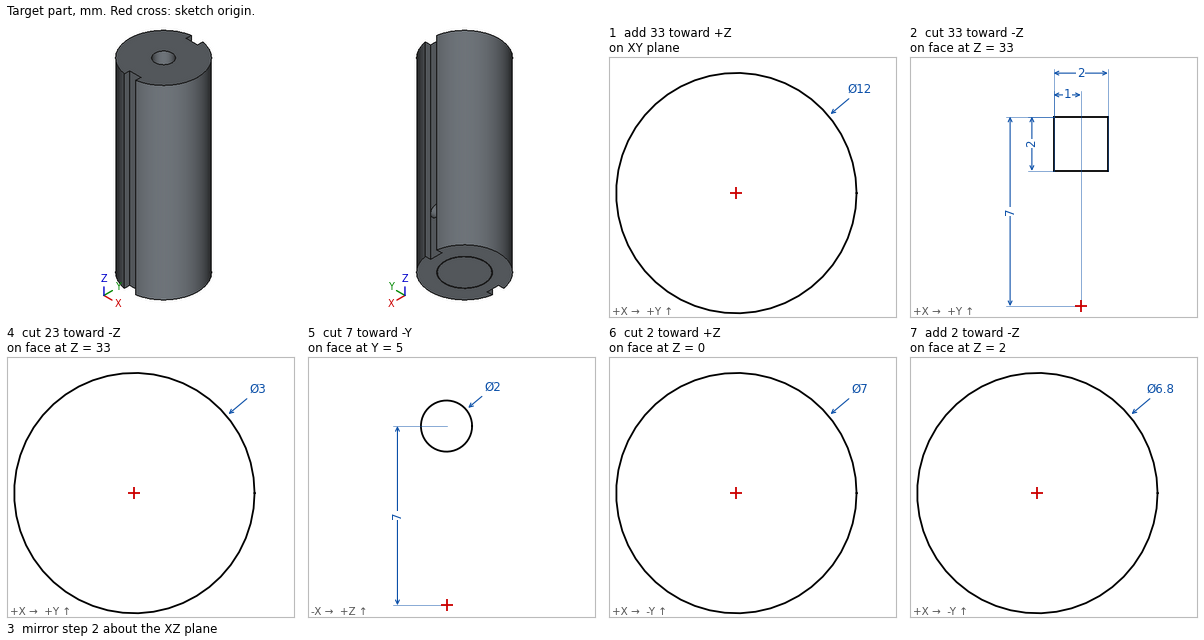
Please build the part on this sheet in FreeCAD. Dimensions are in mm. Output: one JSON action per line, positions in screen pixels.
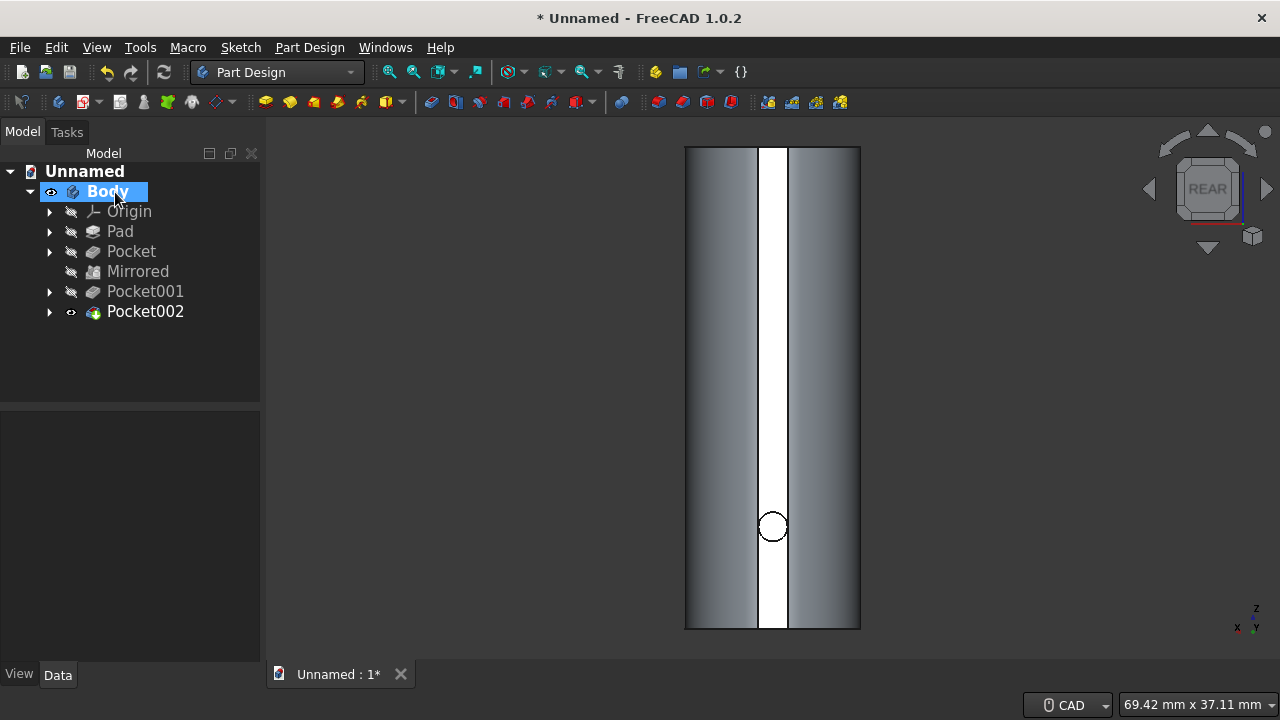
{"action": "key", "text": "5"}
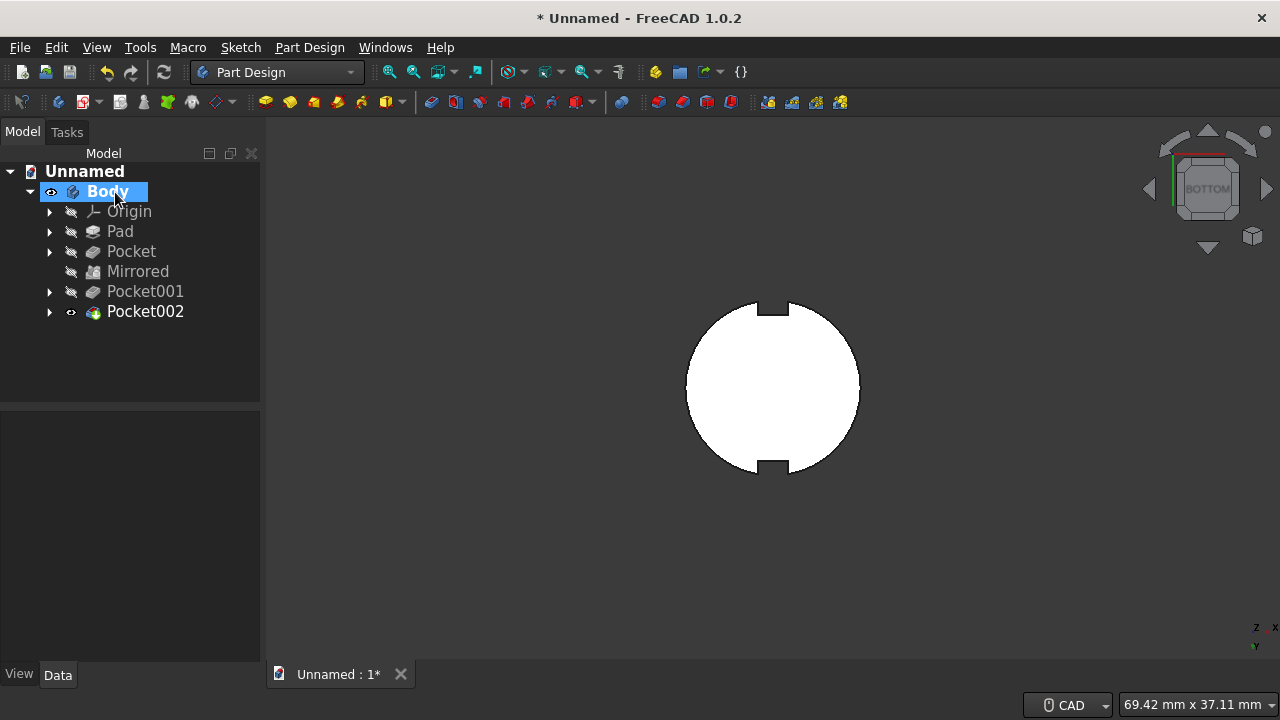
{"action": "key", "text": "v f"}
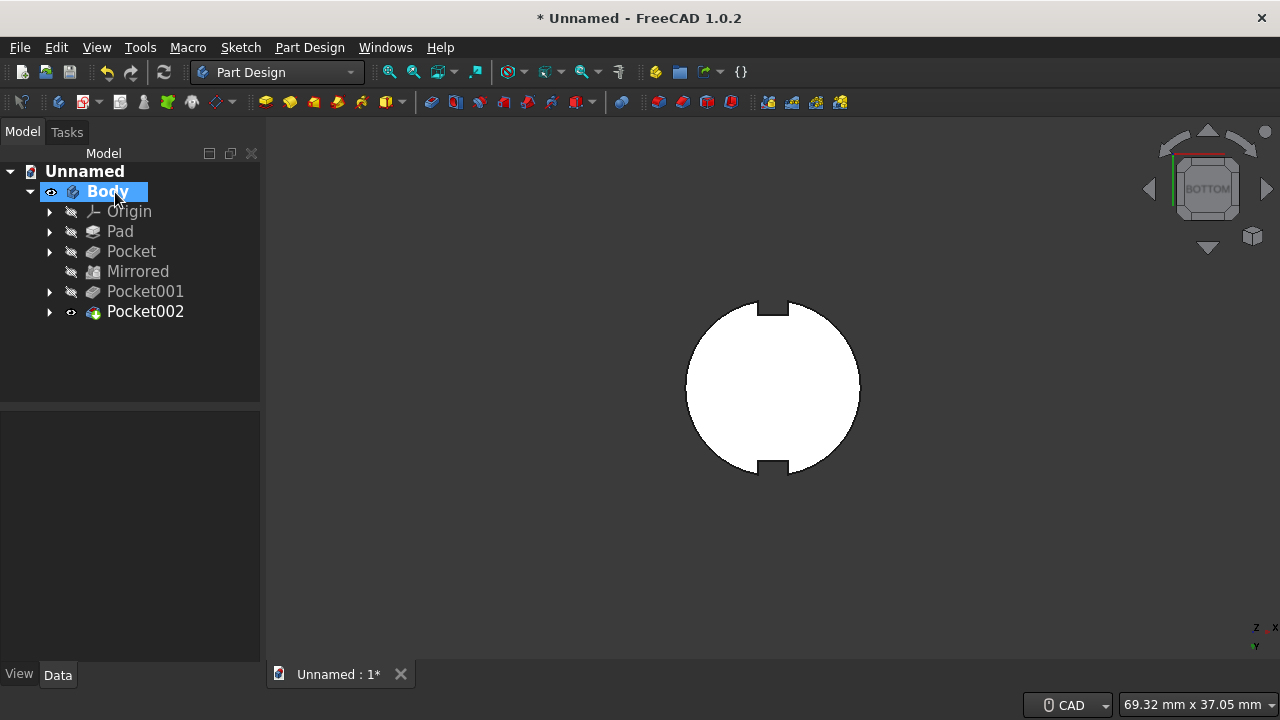
{"action": "left_click", "coordinate": [773, 387]}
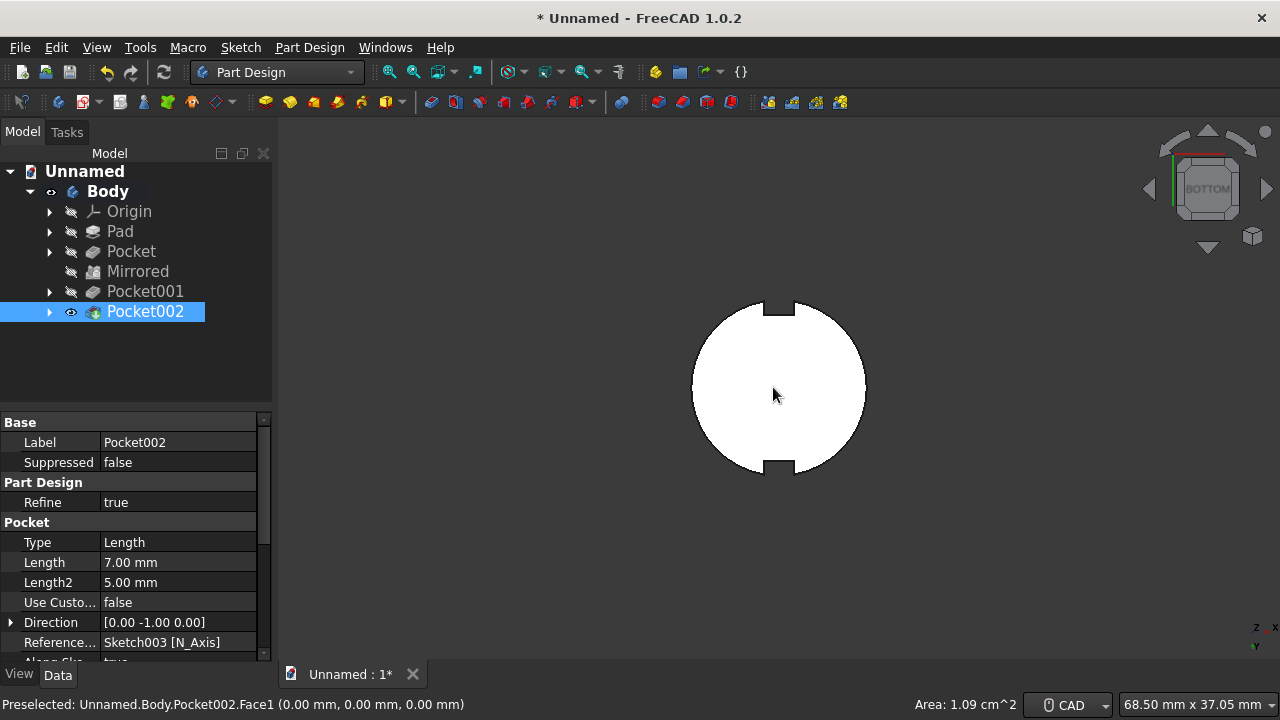
{"action": "left_click", "coordinate": [84, 102]}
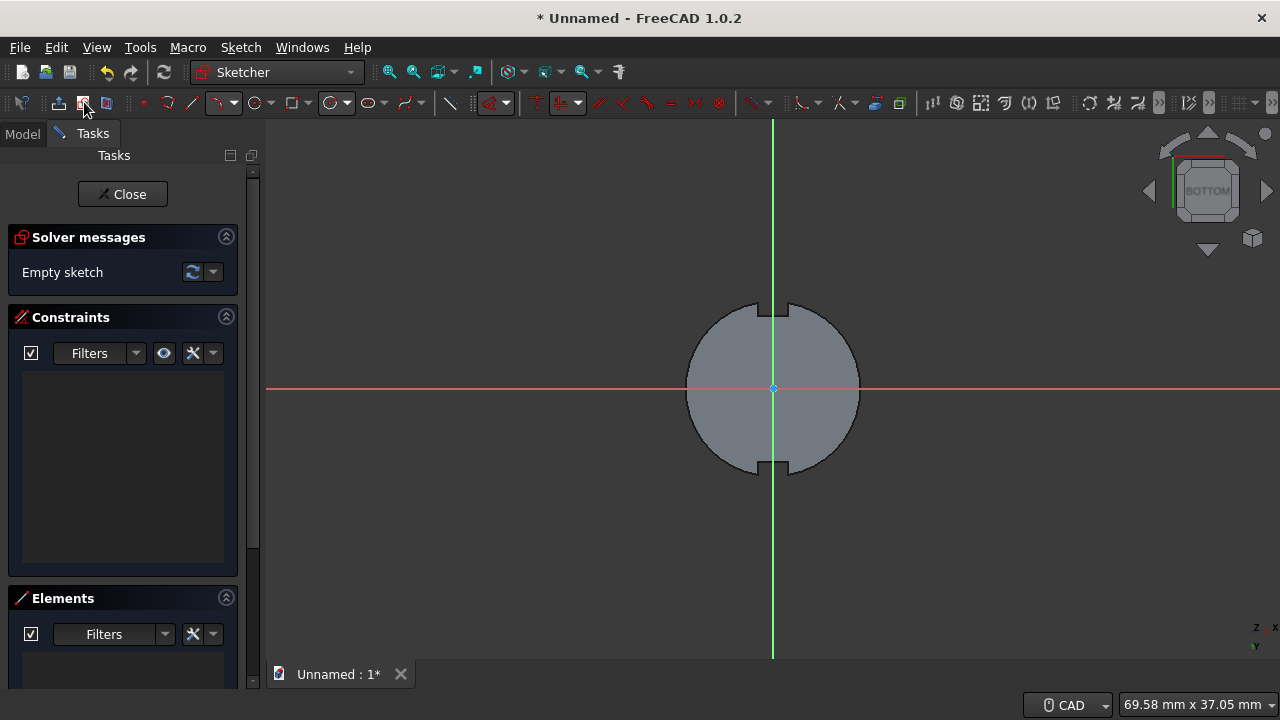
{"action": "scroll", "coordinate": [803, 389], "scroll_direction": "up", "scroll_amount": 6}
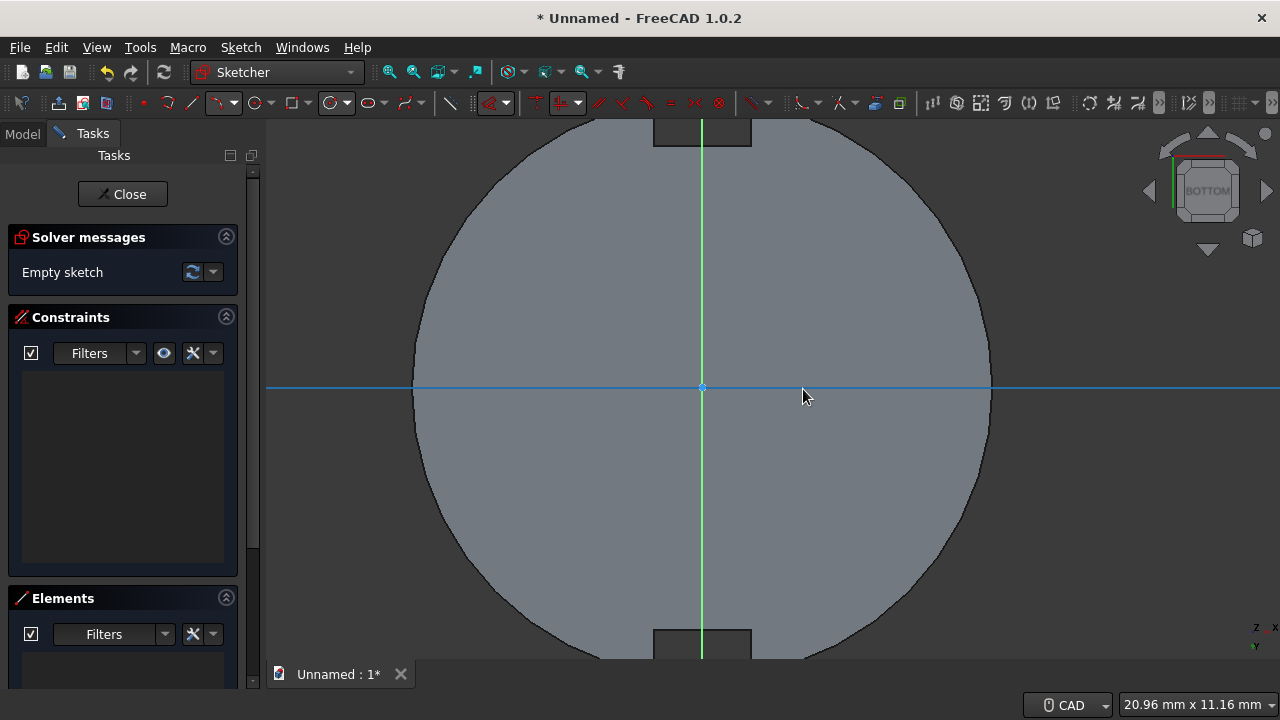
{"action": "left_click", "coordinate": [256, 104]}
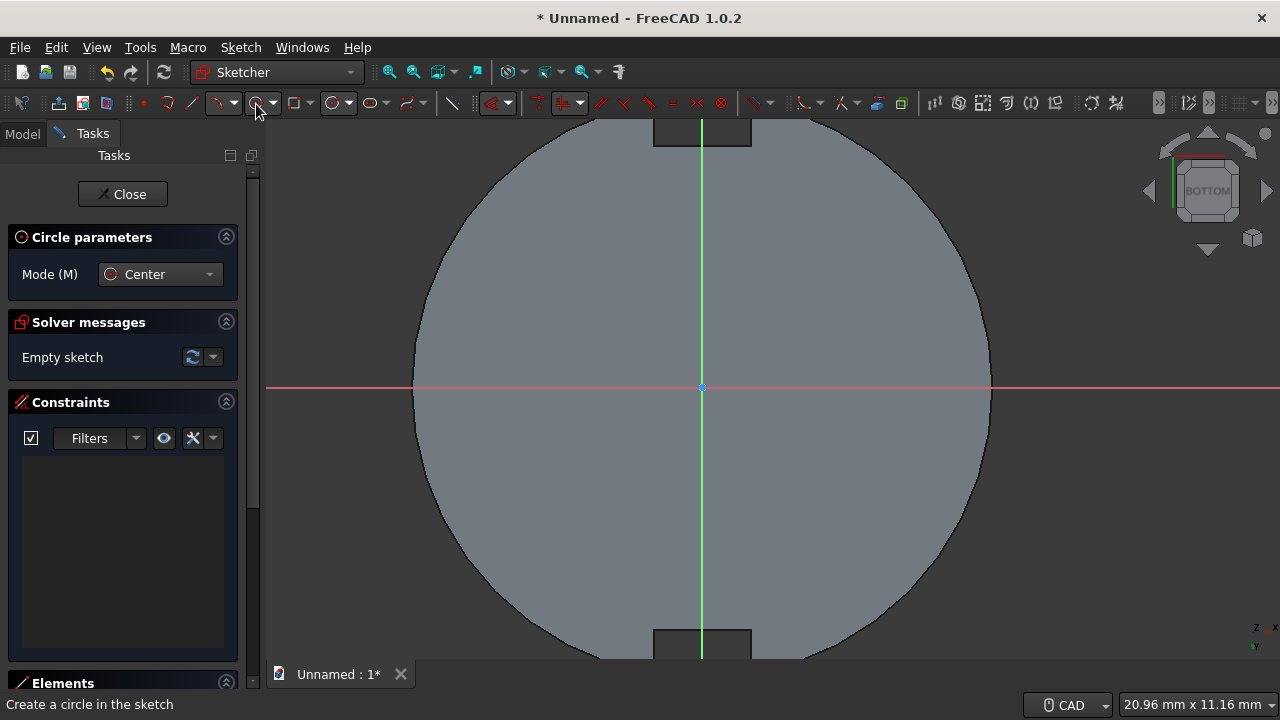
{"action": "left_click", "coordinate": [702, 388]}
{"action": "left_click", "coordinate": [822, 268]}
{"action": "key", "text": "Escape"}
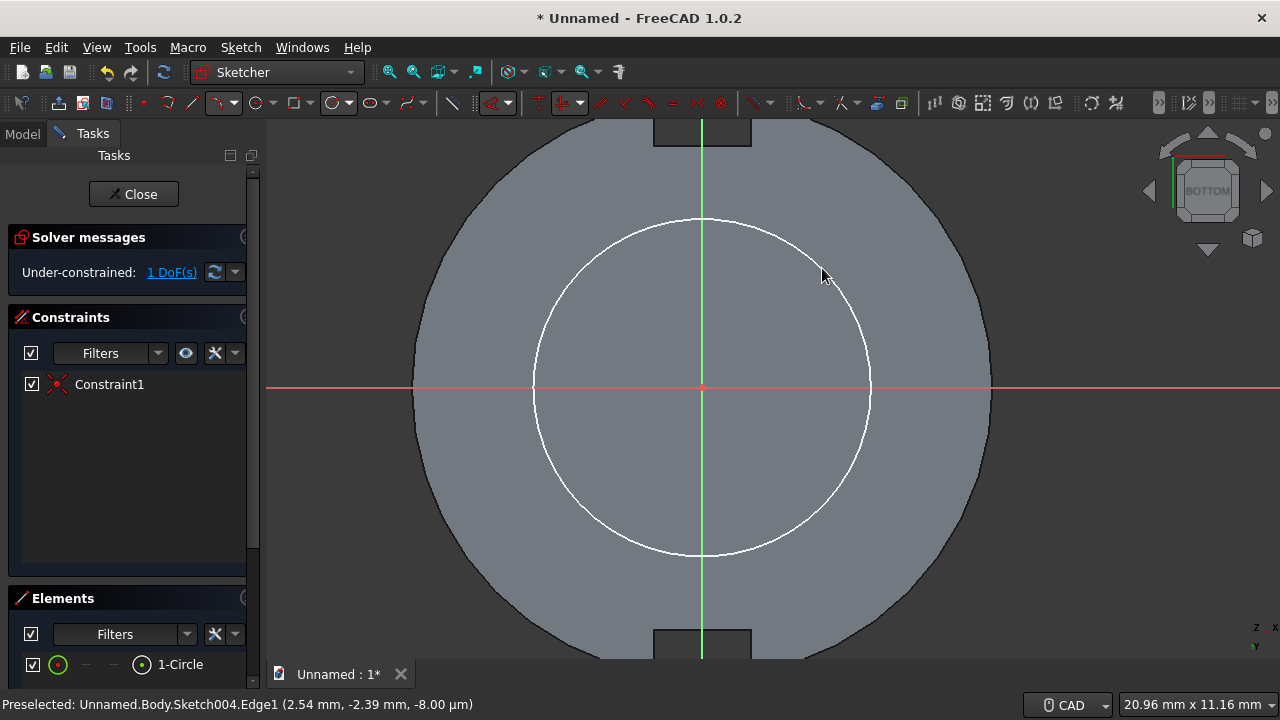
{"action": "key", "text": "d"}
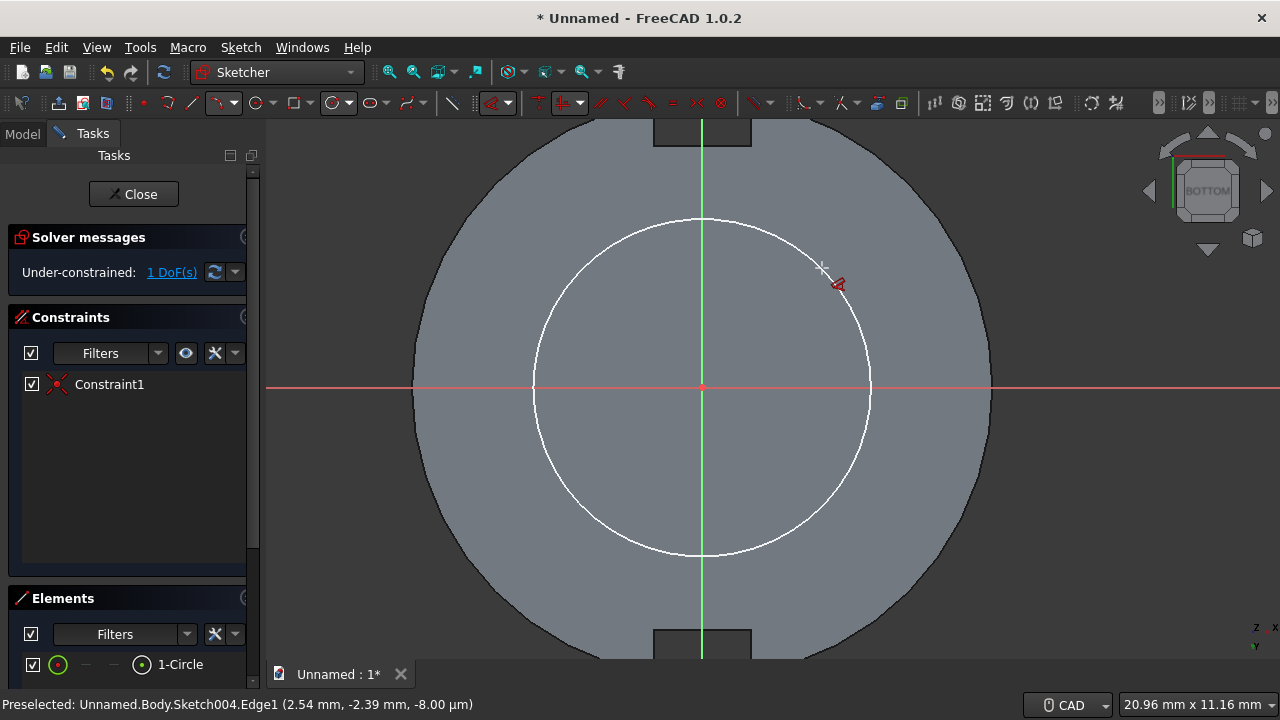
{"action": "left_click", "coordinate": [821, 268]}
{"action": "left_click", "coordinate": [844, 245]}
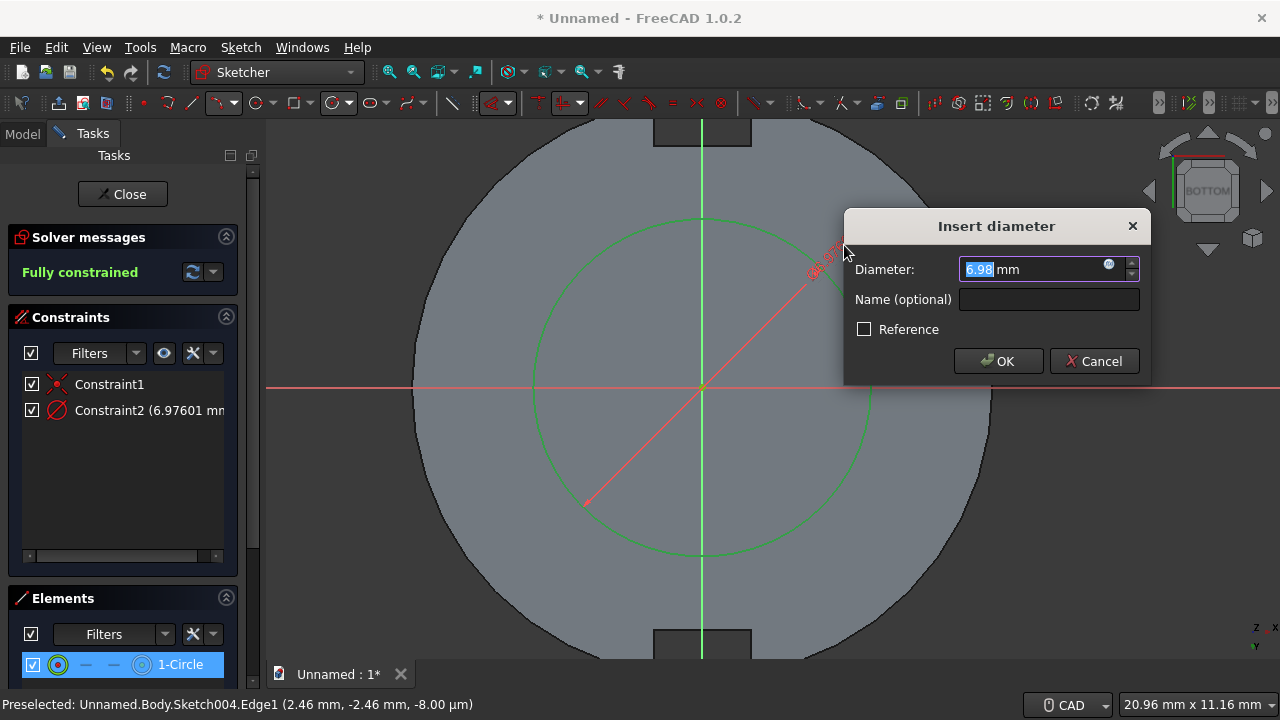
{"action": "type", "text": "7"}
{"action": "key", "text": "Return"}
{"action": "key", "text": "Escape"}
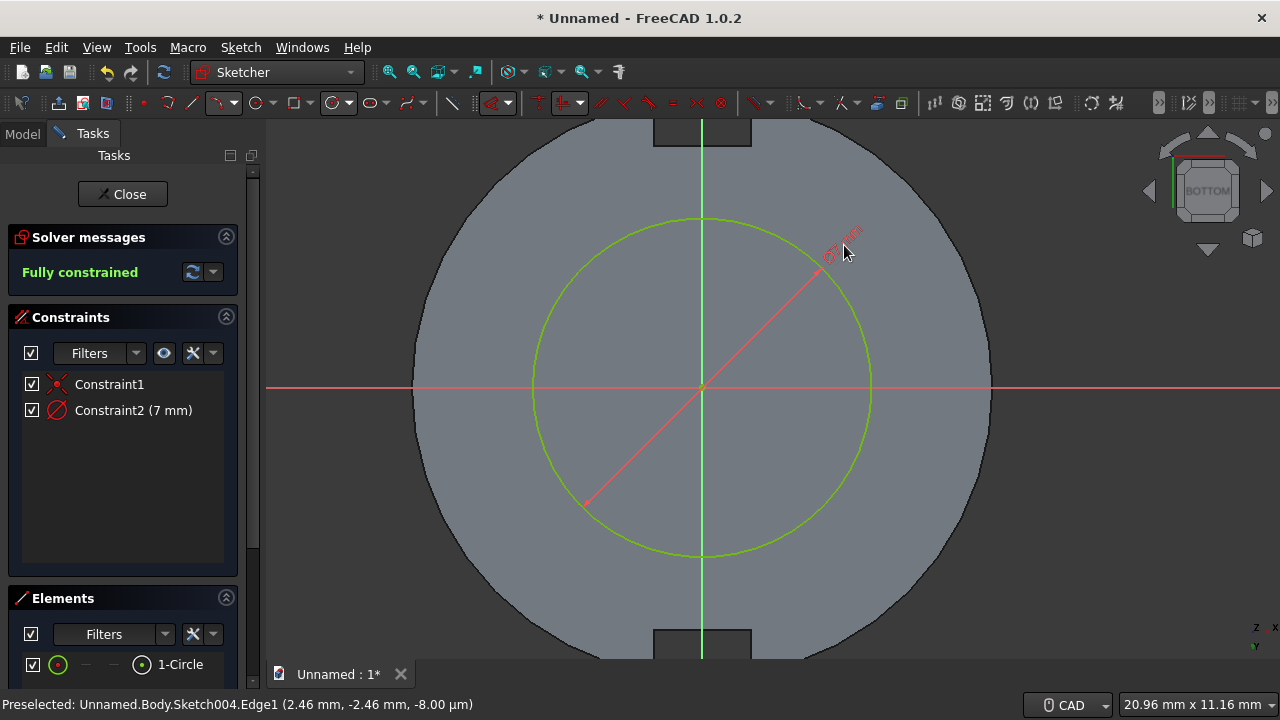
{"action": "left_click", "coordinate": [123, 194]}